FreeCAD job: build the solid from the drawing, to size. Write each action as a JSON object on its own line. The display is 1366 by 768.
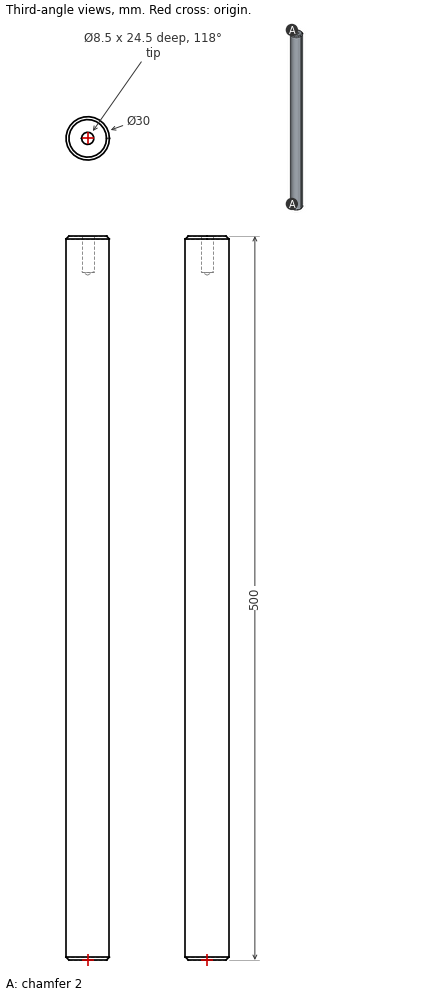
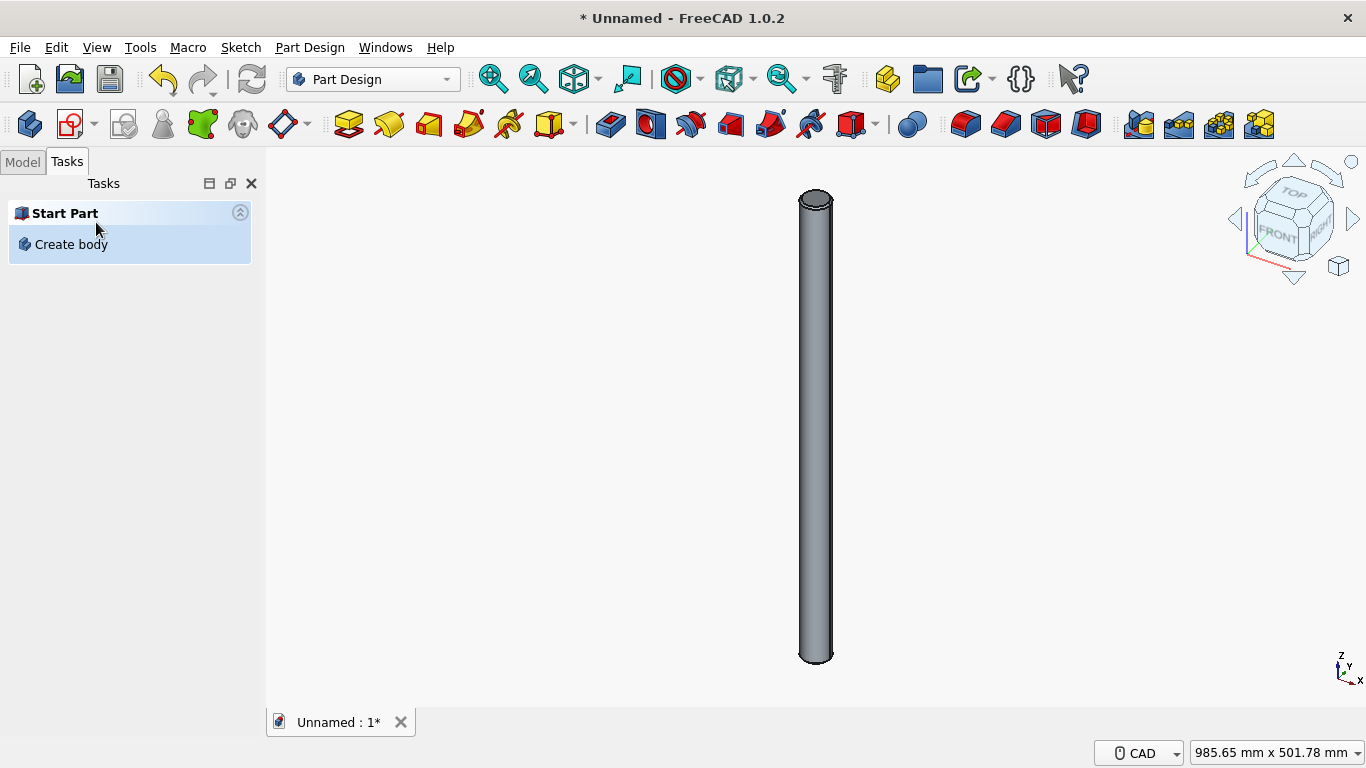
{"action": "left_click", "coordinate": [816, 197]}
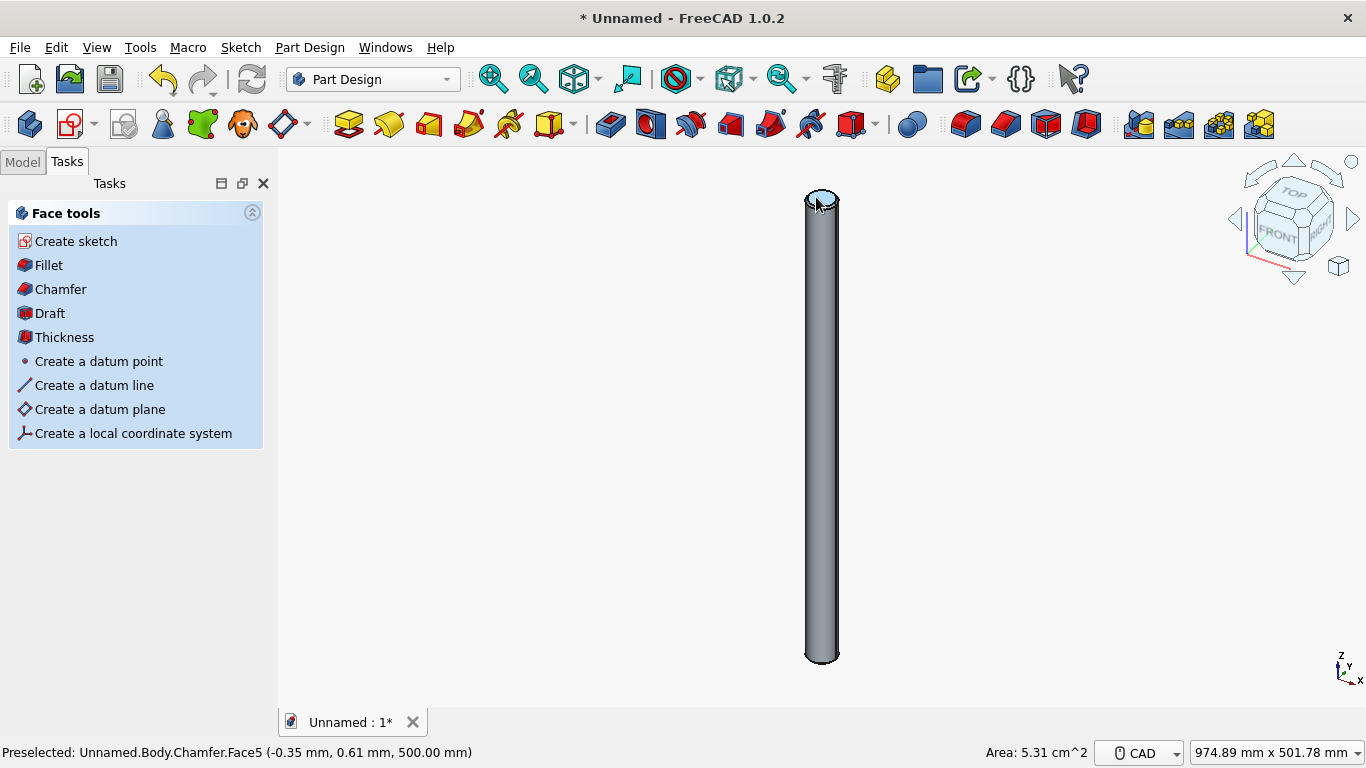
{"action": "left_click", "coordinate": [70, 124]}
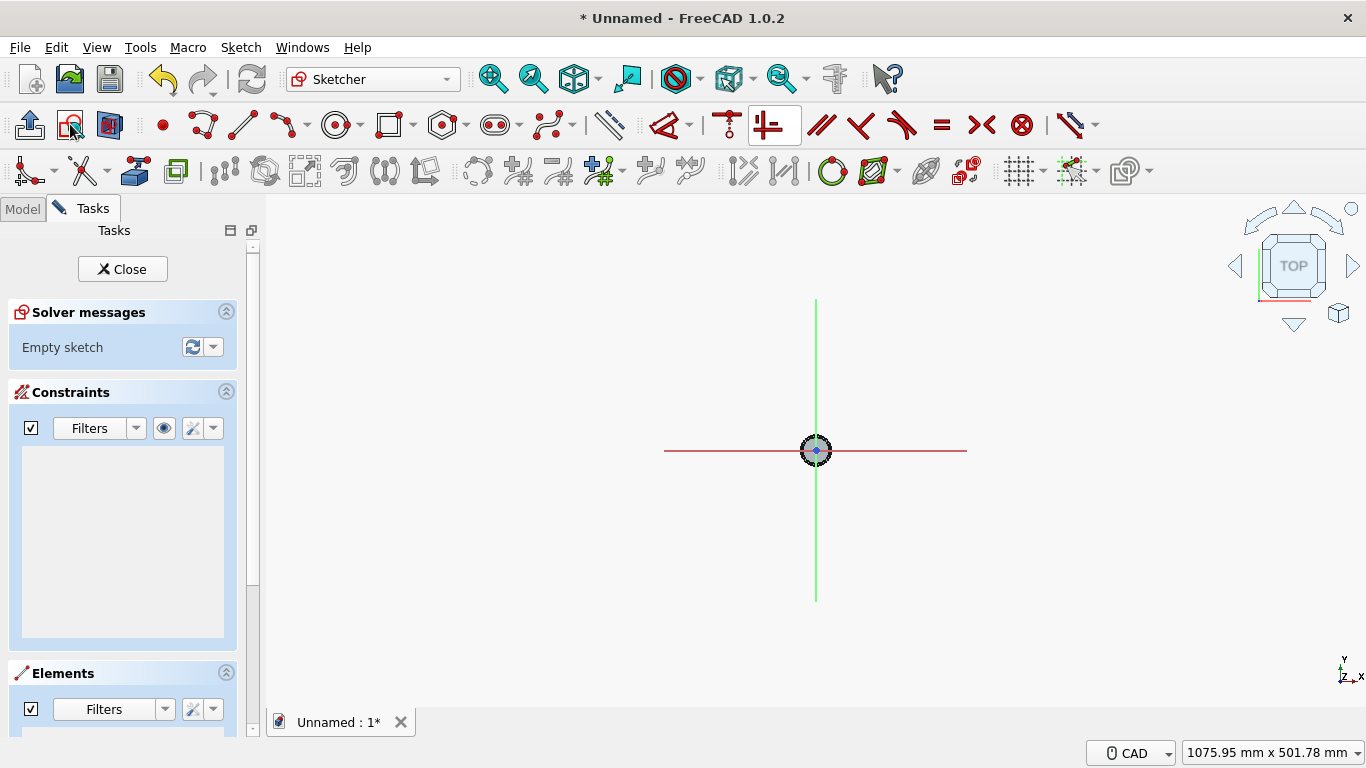
{"action": "scroll", "coordinate": [820, 451], "scroll_direction": "up", "scroll_amount": 15}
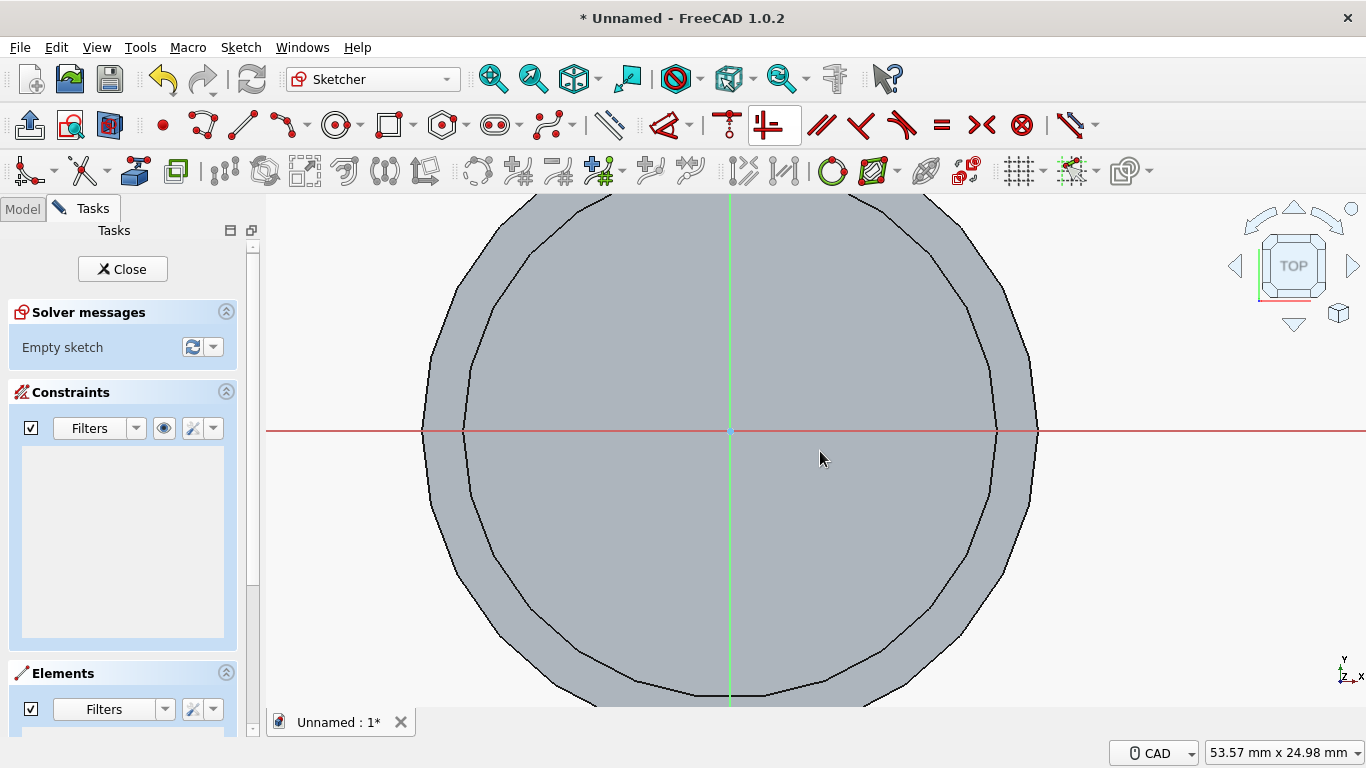
{"action": "scroll", "coordinate": [709, 408], "scroll_direction": "up", "scroll_amount": 3}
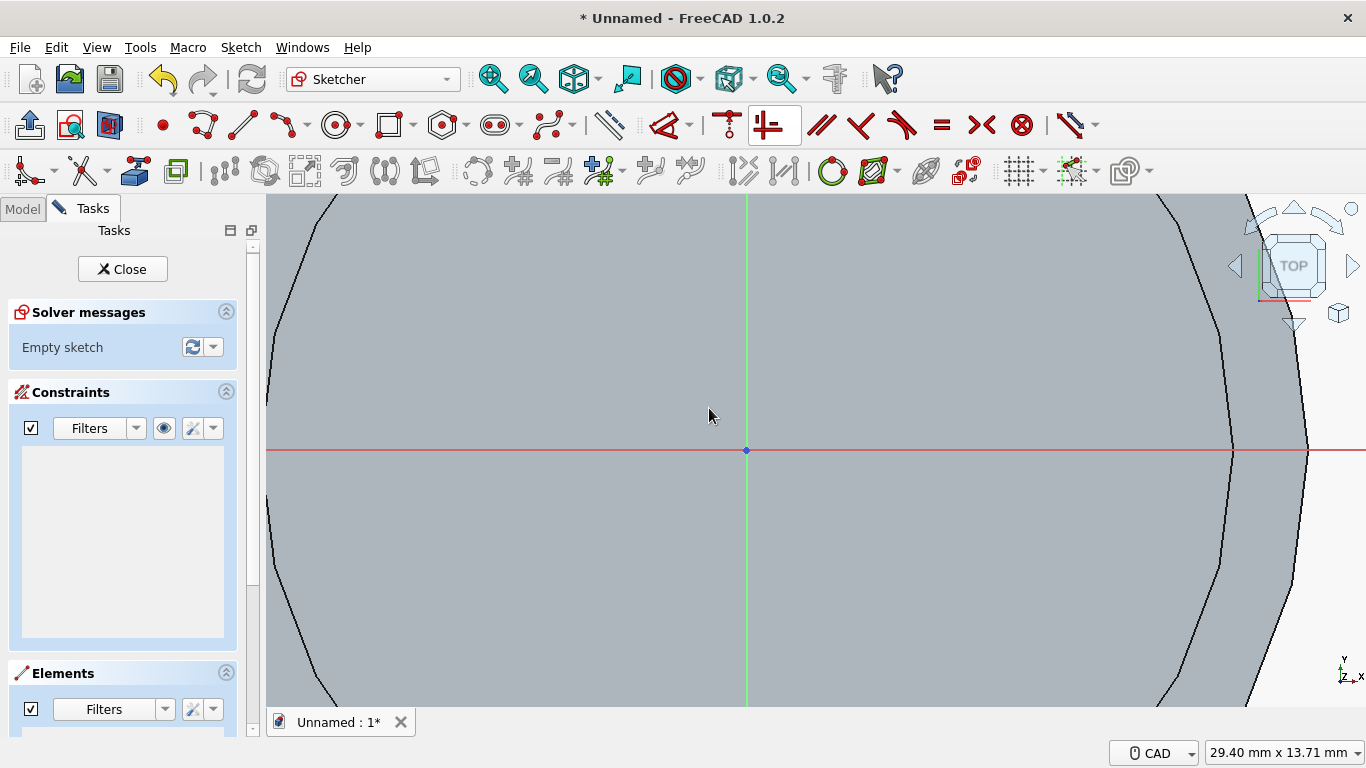
{"action": "key", "text": "g c"}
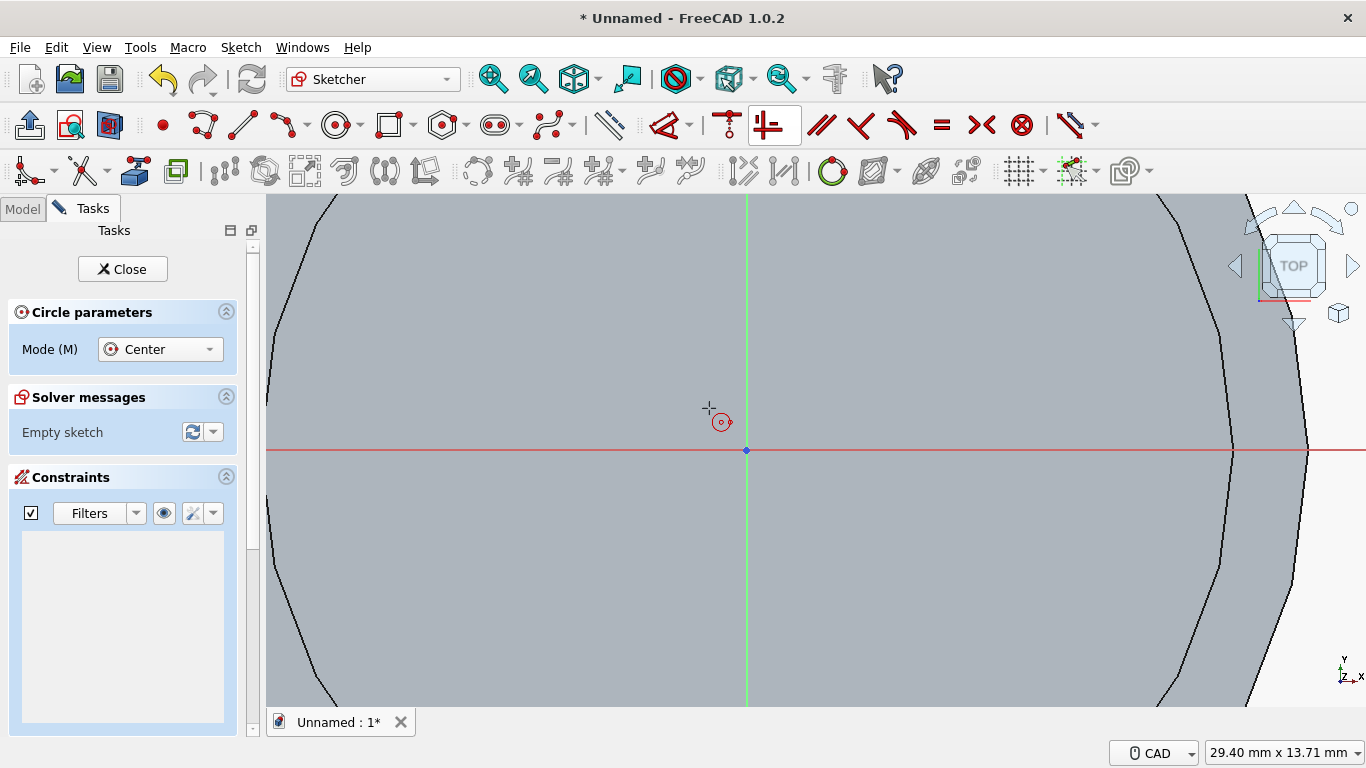
{"action": "left_click", "coordinate": [747, 450]}
{"action": "left_click", "coordinate": [859, 338]}
{"action": "key", "text": "Escape"}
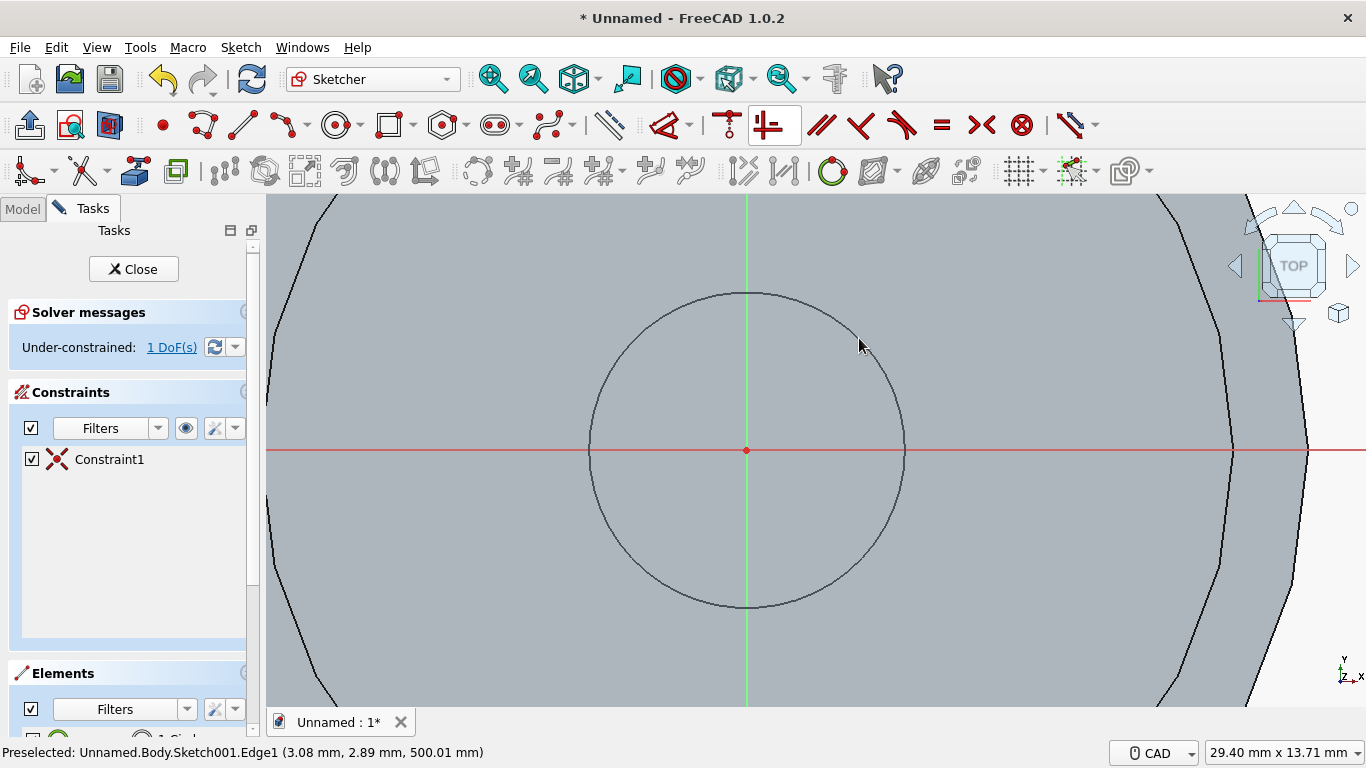
{"action": "key", "text": "d"}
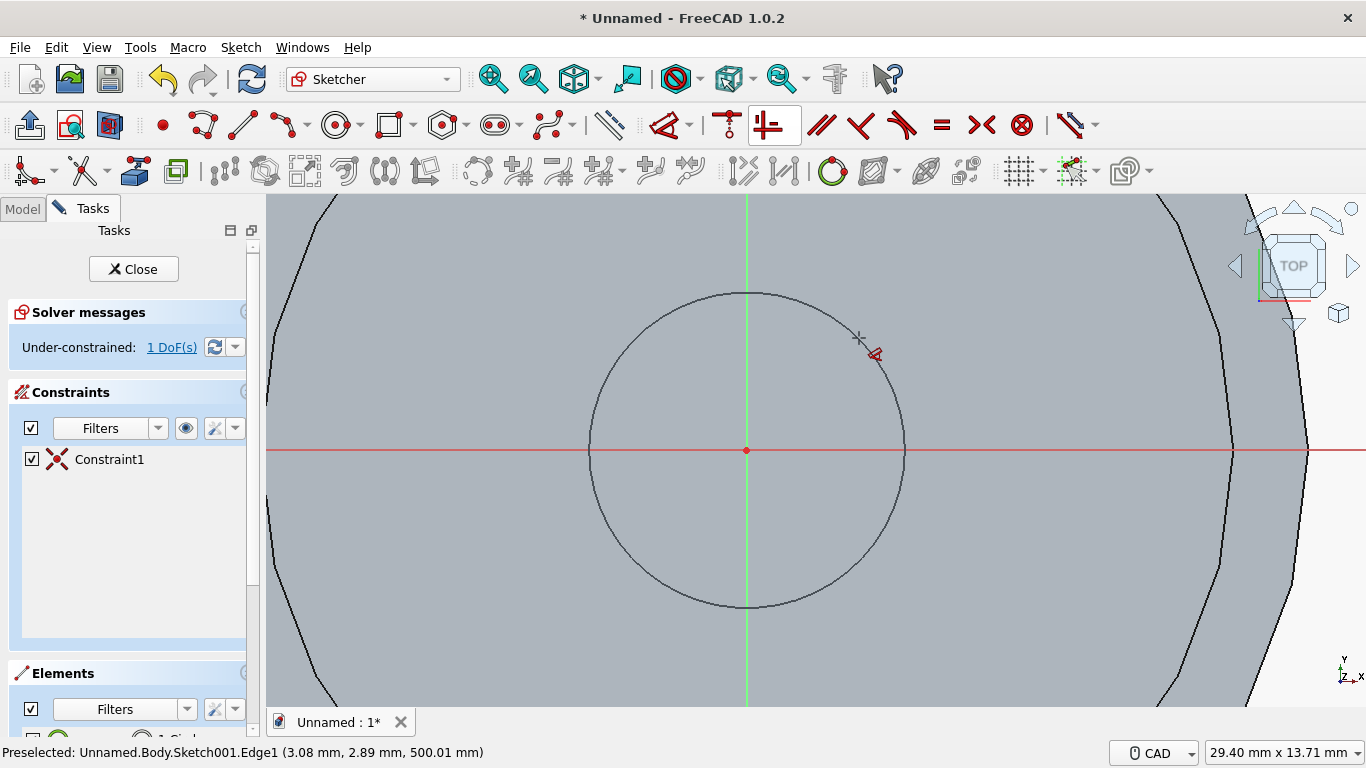
{"action": "left_click", "coordinate": [858, 338]}
{"action": "left_click", "coordinate": [881, 315]}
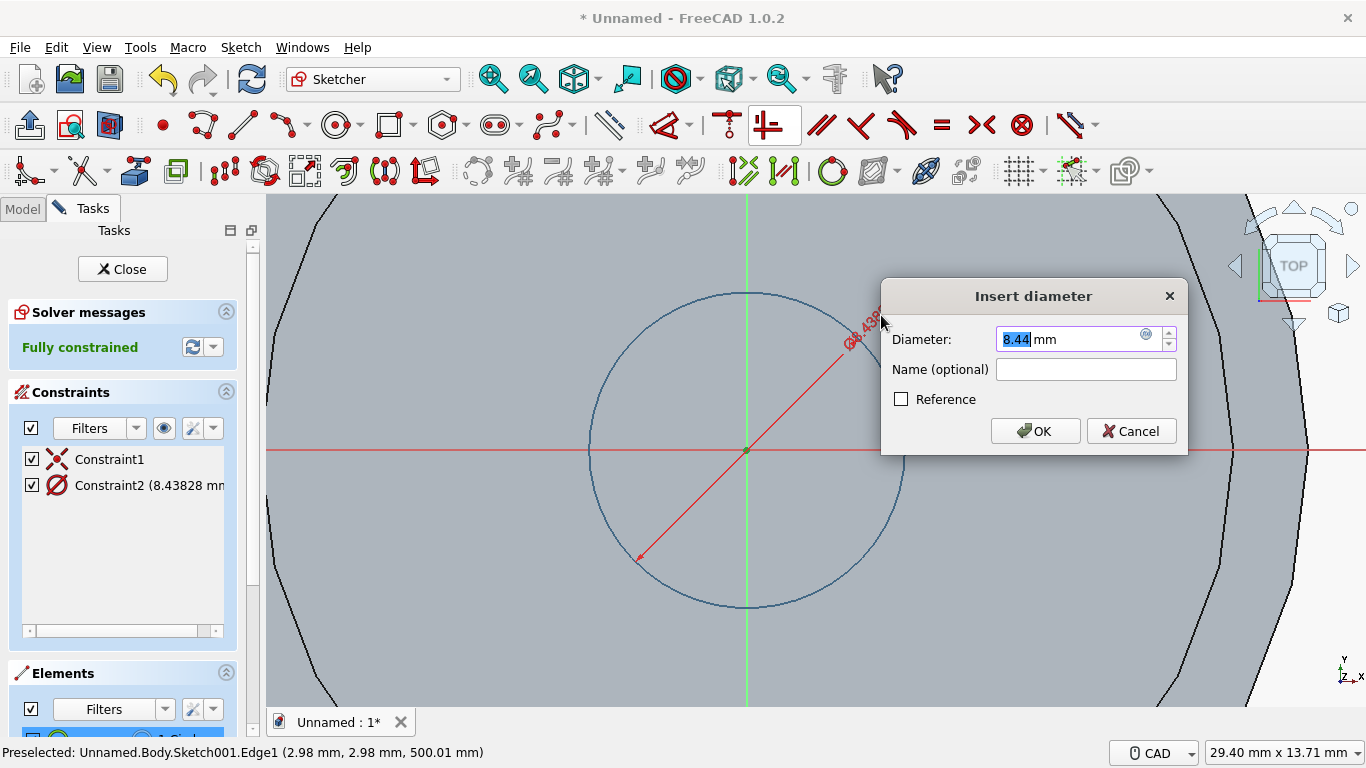
{"action": "type", "text": "8.5"}
{"action": "key", "text": "Return"}
{"action": "key", "text": "Escape"}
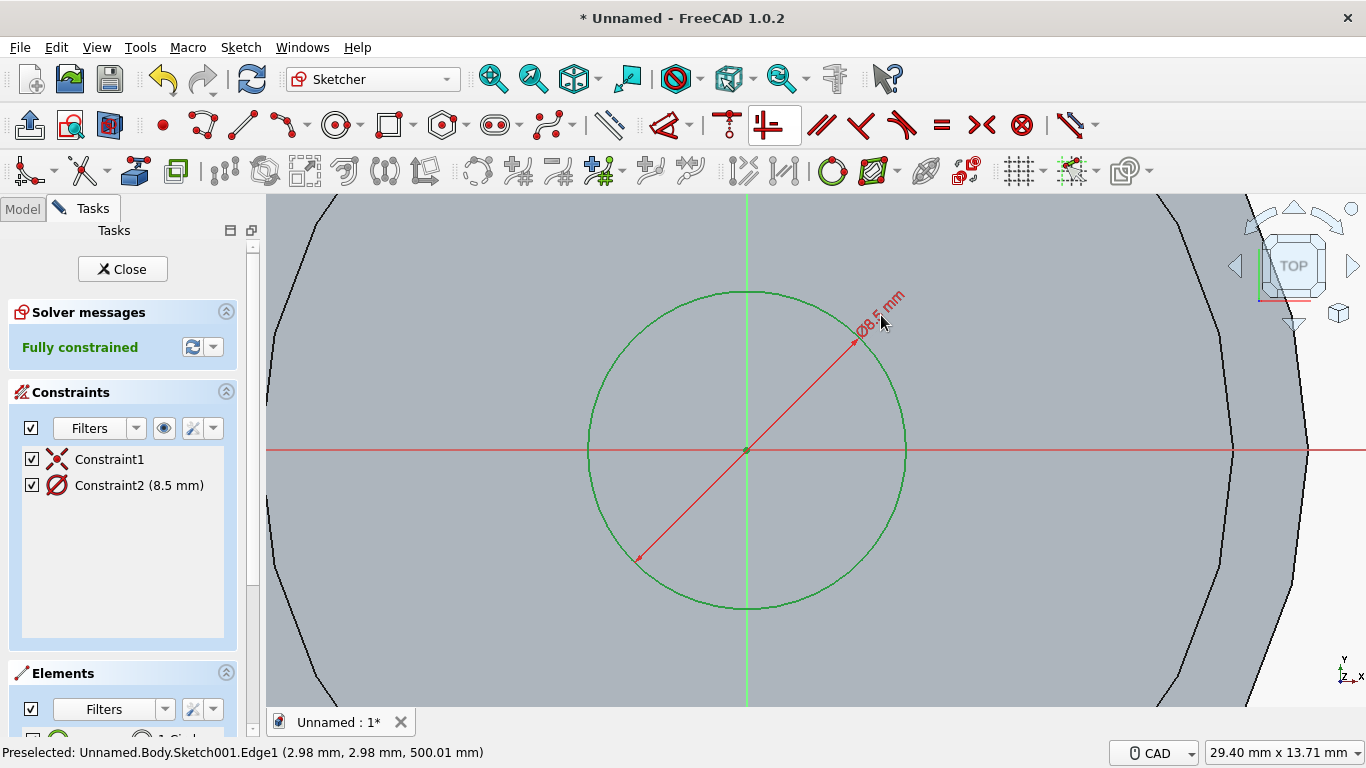
{"action": "left_click", "coordinate": [123, 269]}